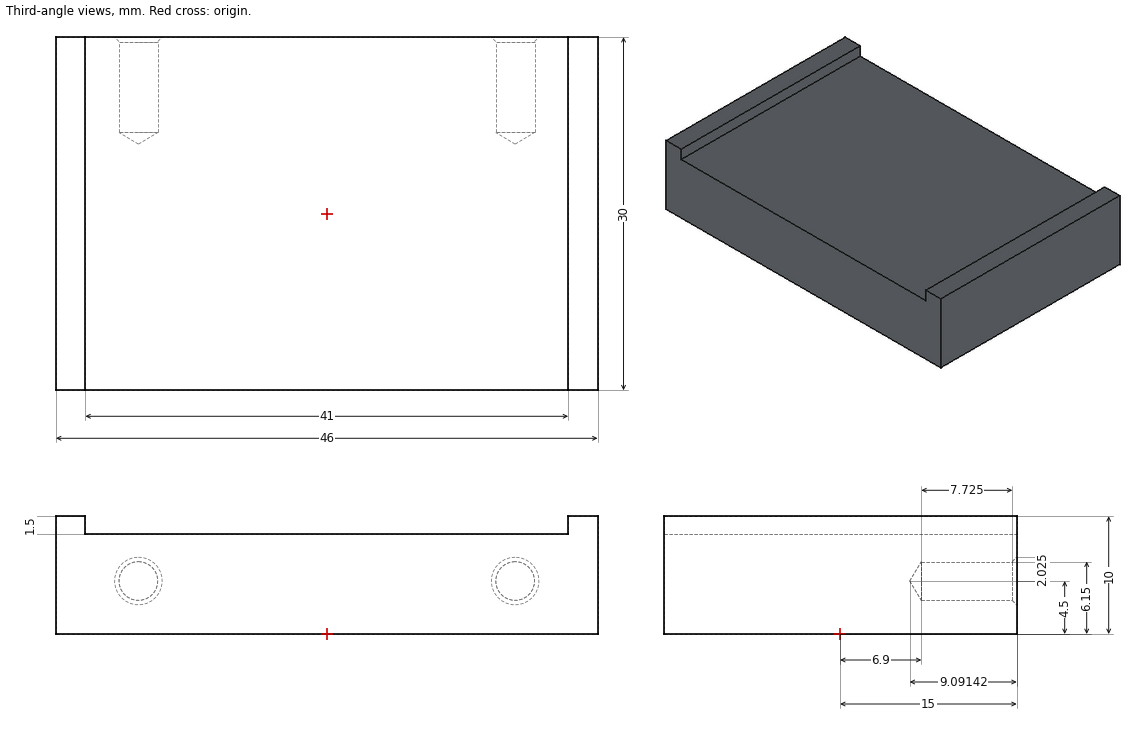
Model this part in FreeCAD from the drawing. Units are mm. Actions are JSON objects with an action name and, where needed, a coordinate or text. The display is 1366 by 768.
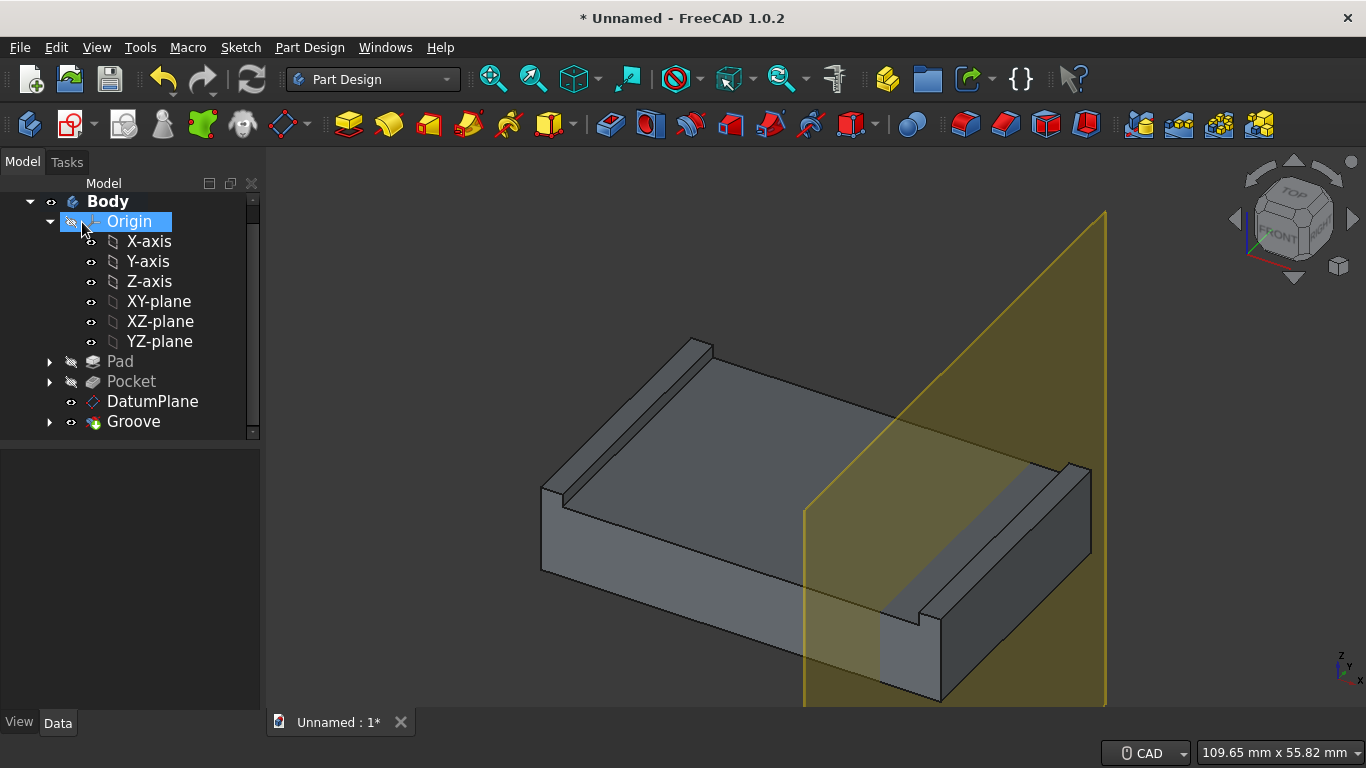
{"action": "left_click", "coordinate": [116, 402]}
{"action": "key", "text": "space"}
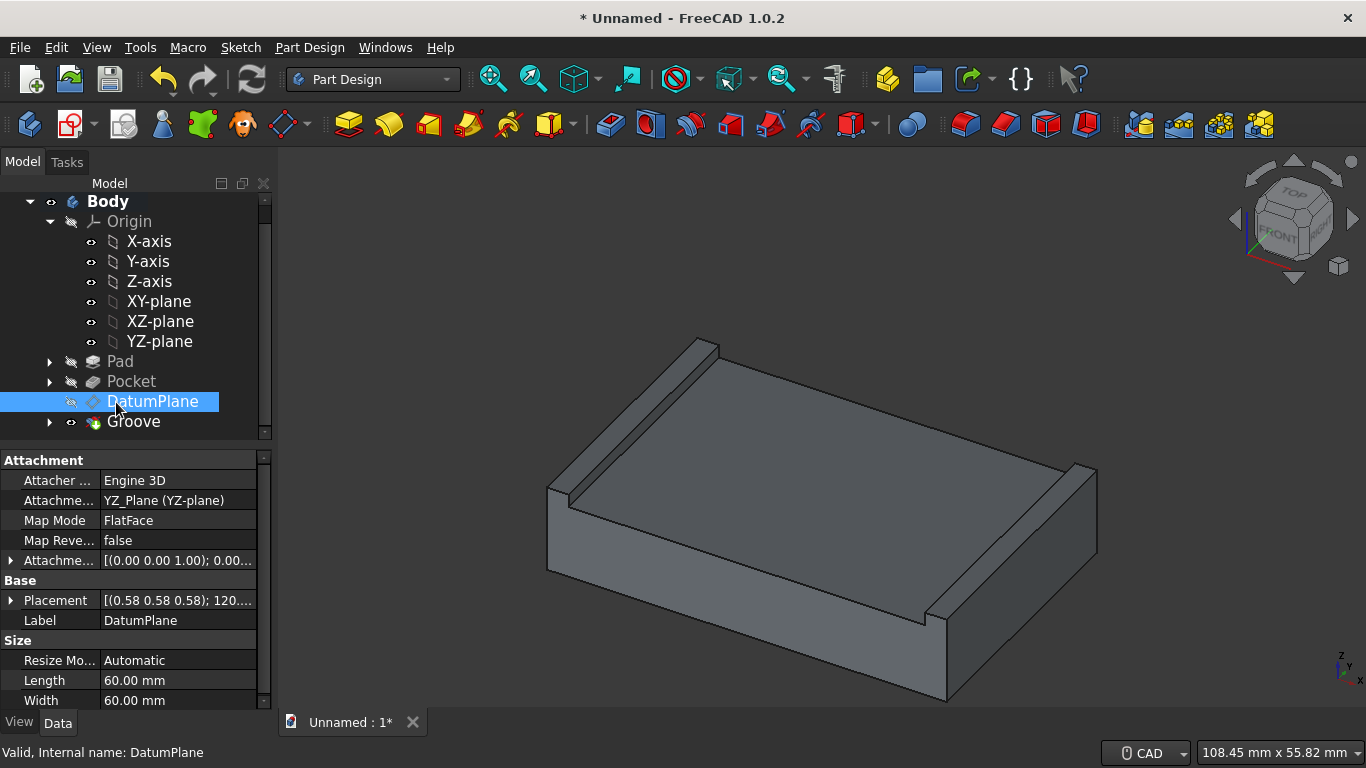
{"action": "left_click", "coordinate": [116, 422]}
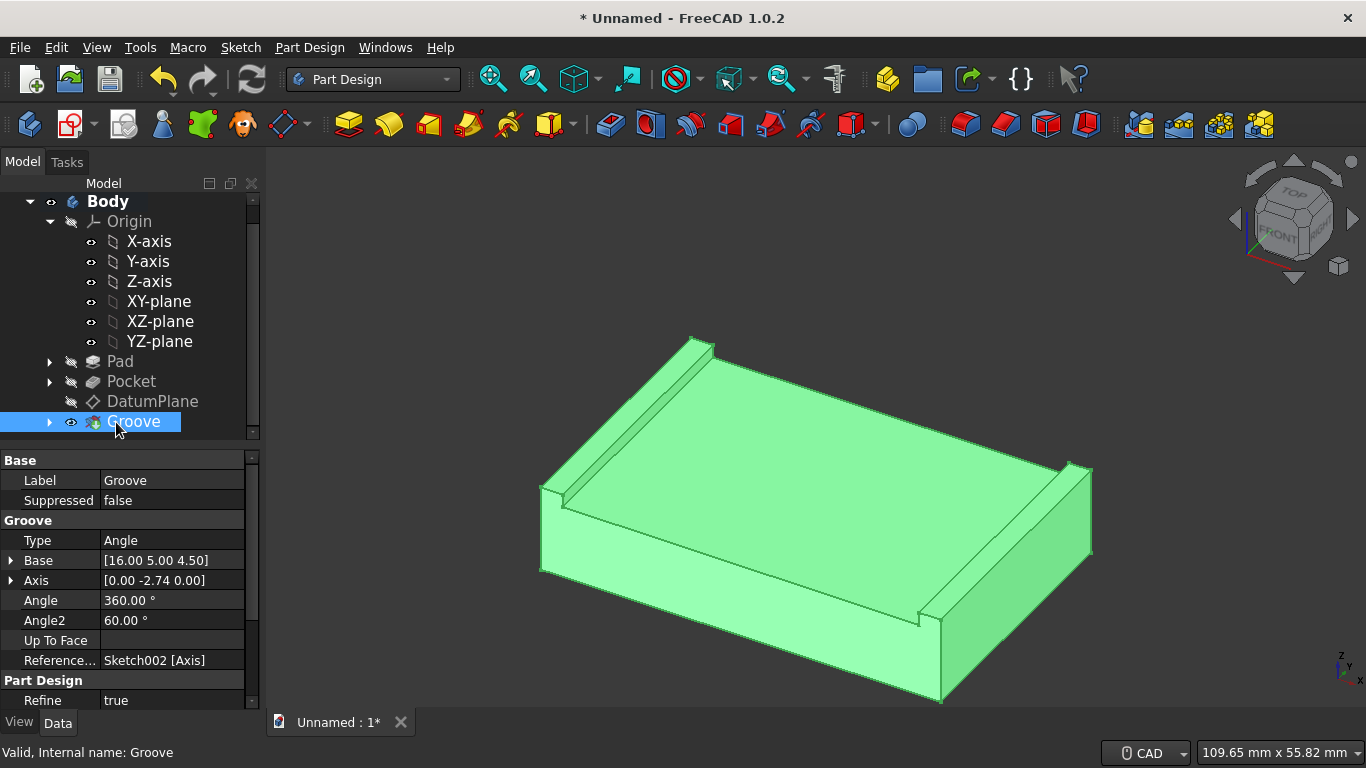
{"action": "left_click", "coordinate": [1140, 124]}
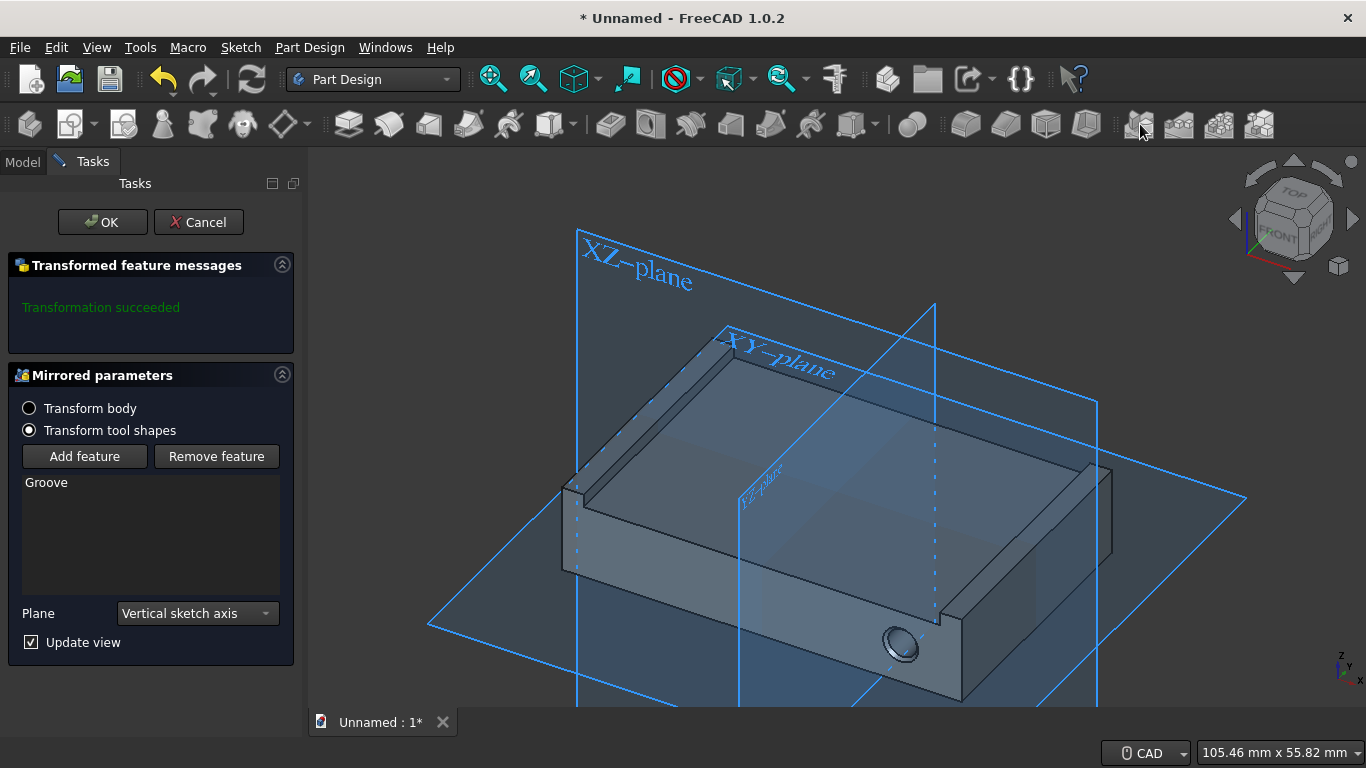
{"action": "left_click", "coordinate": [198, 614]}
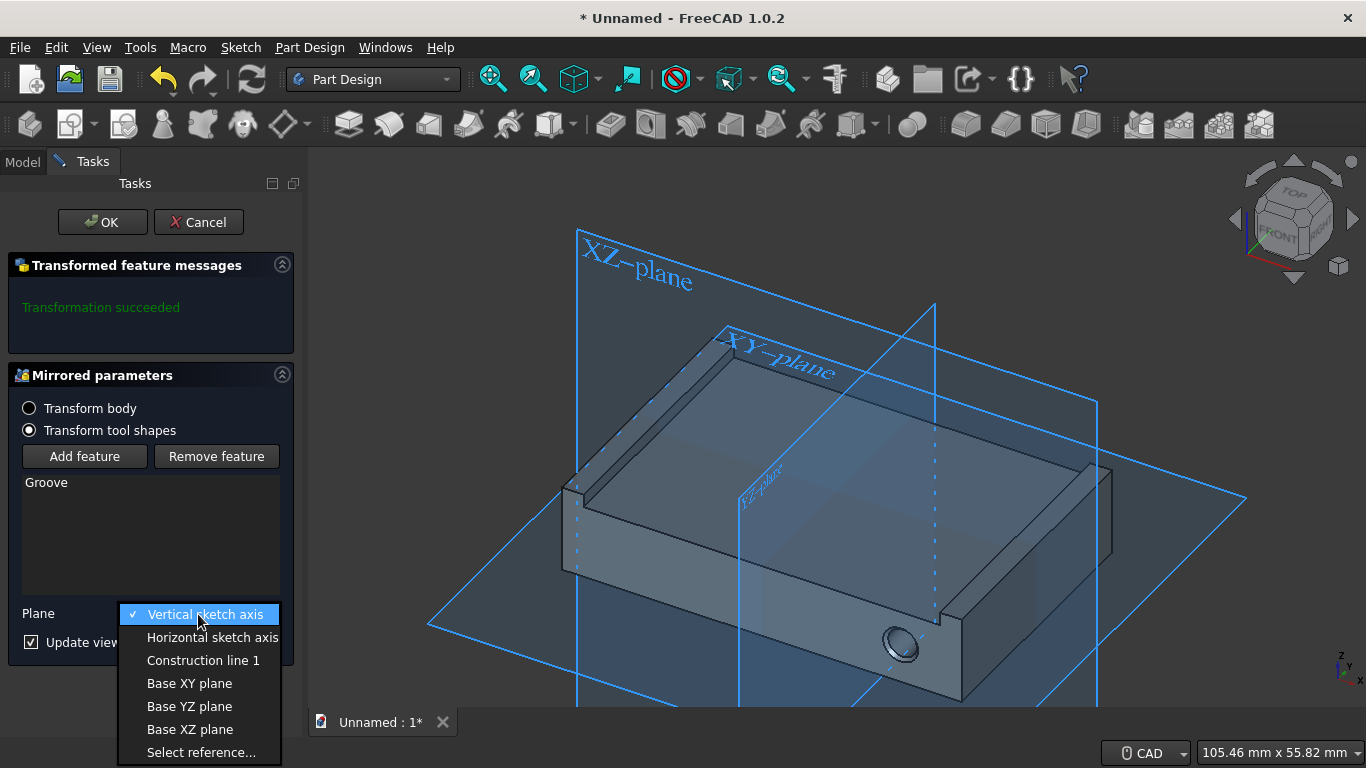
{"action": "left_click", "coordinate": [198, 706]}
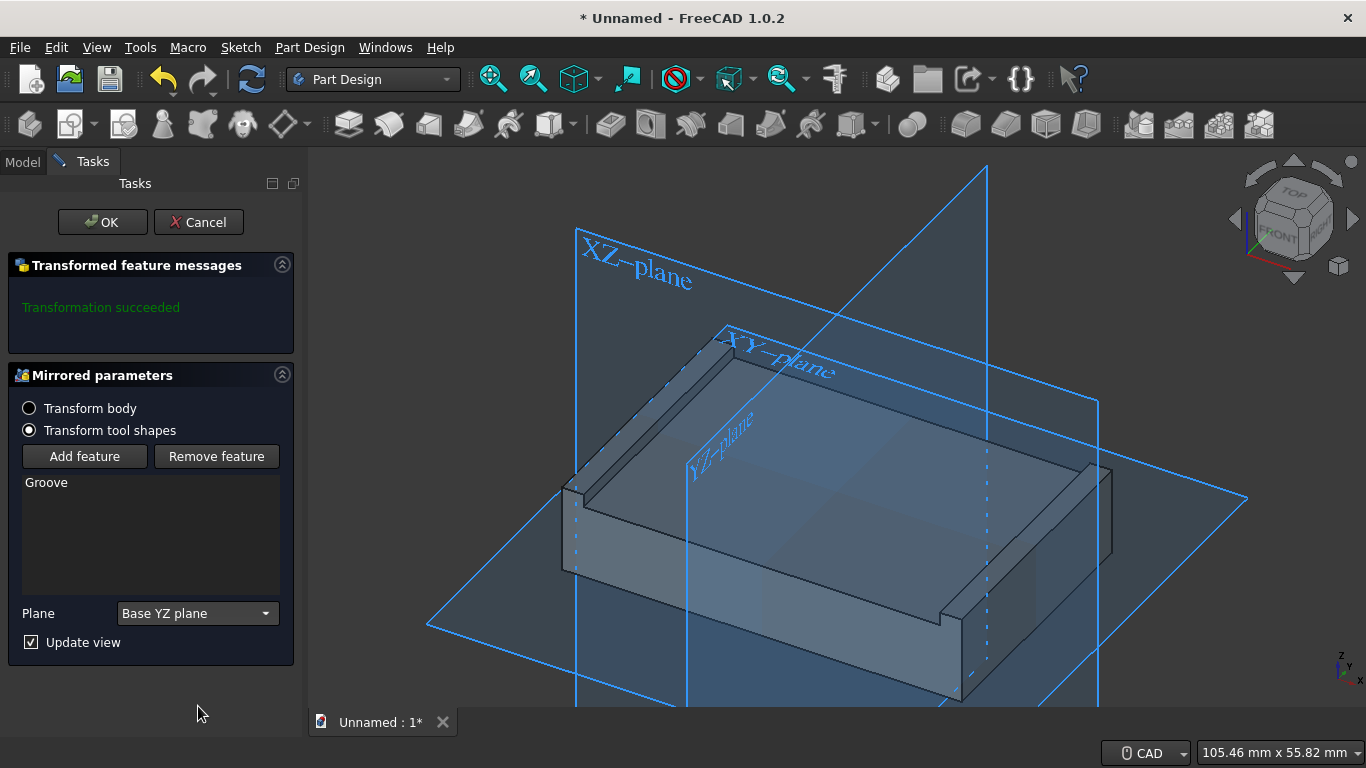
{"action": "left_click", "coordinate": [103, 222]}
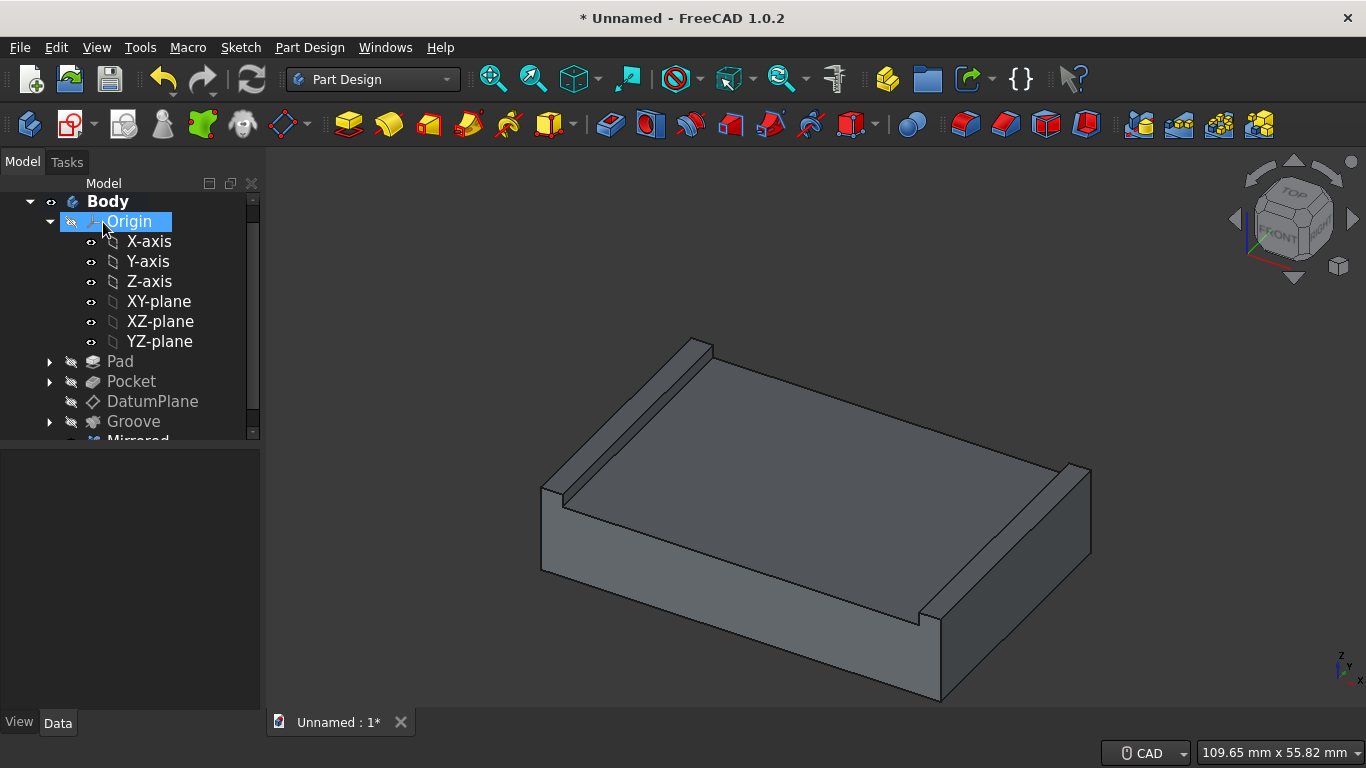
{"action": "key", "text": "0"}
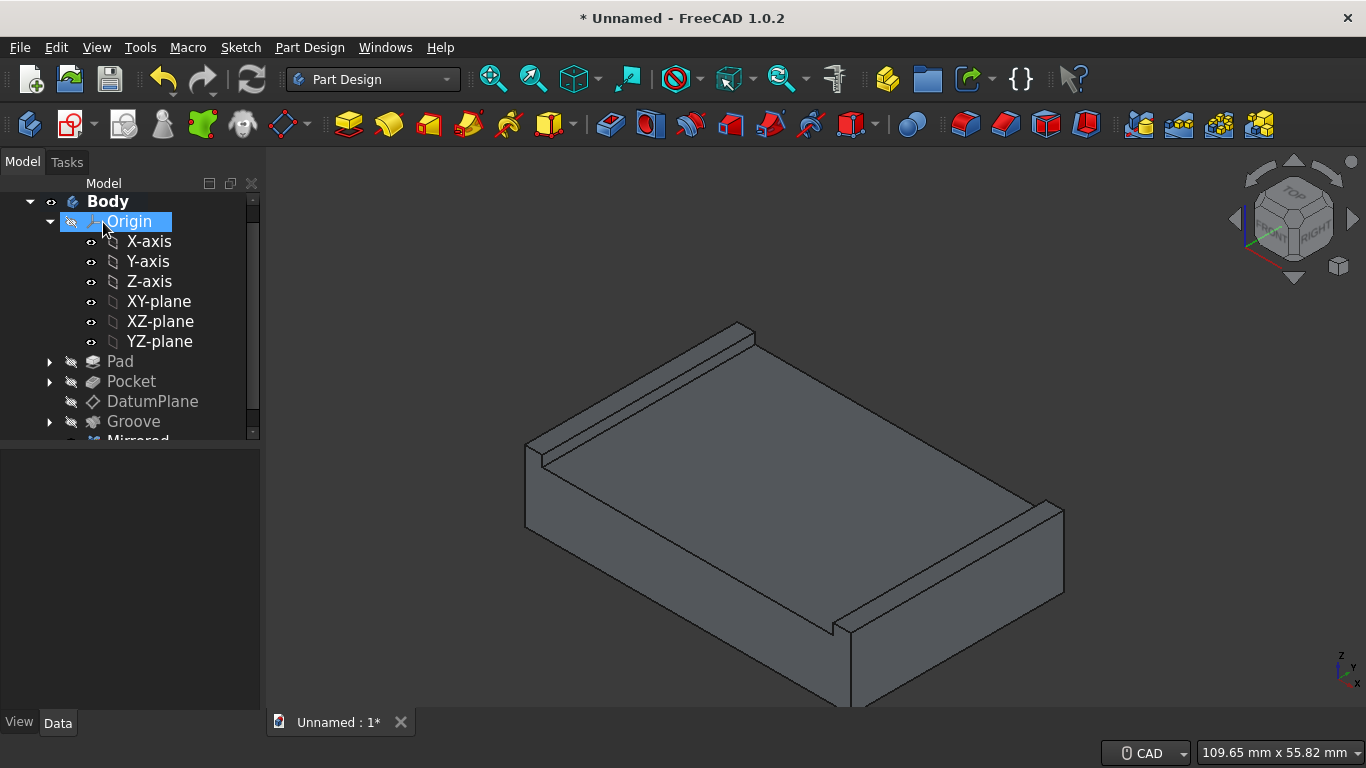
{"action": "key", "text": "v f"}